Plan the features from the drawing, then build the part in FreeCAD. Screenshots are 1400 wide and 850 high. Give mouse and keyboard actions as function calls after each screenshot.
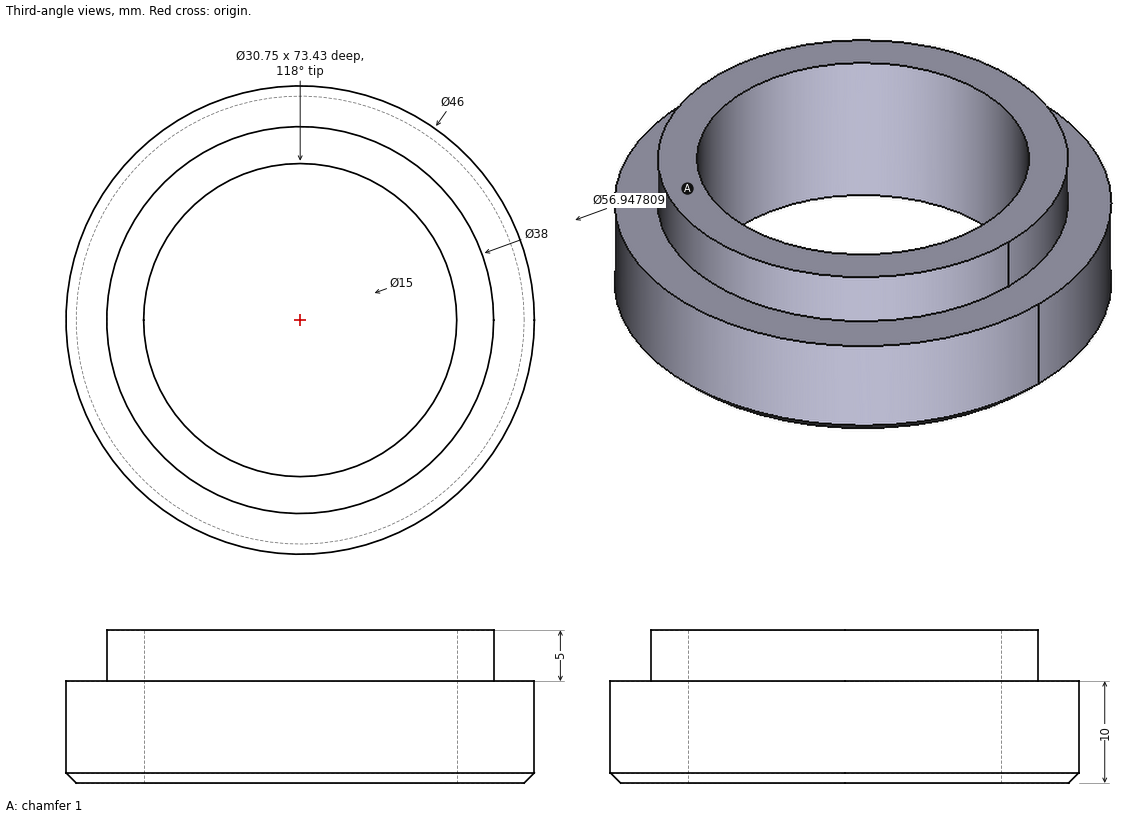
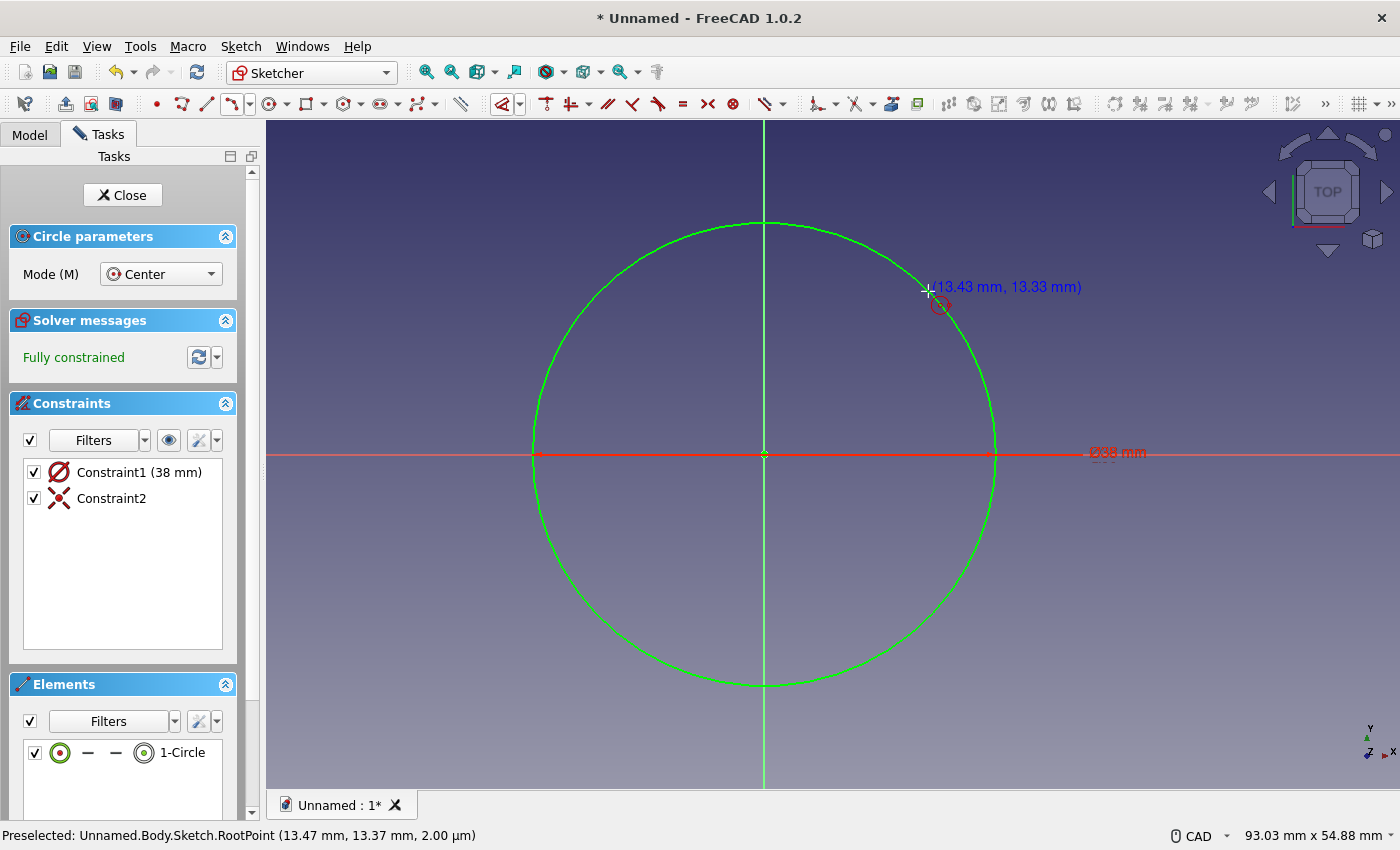
click(764, 454)
move(829, 390)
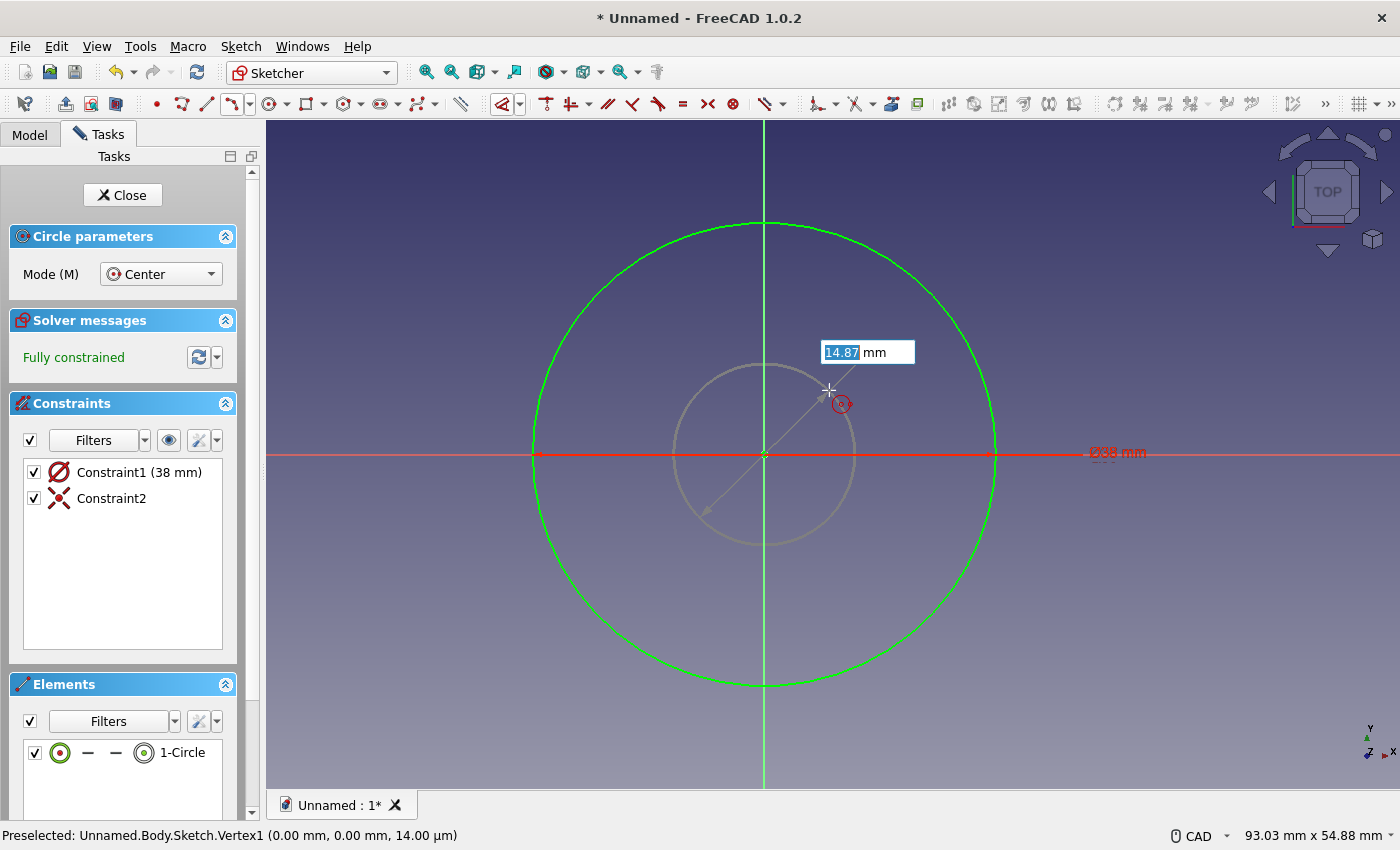
text(15)
key(Return)
key(Escape)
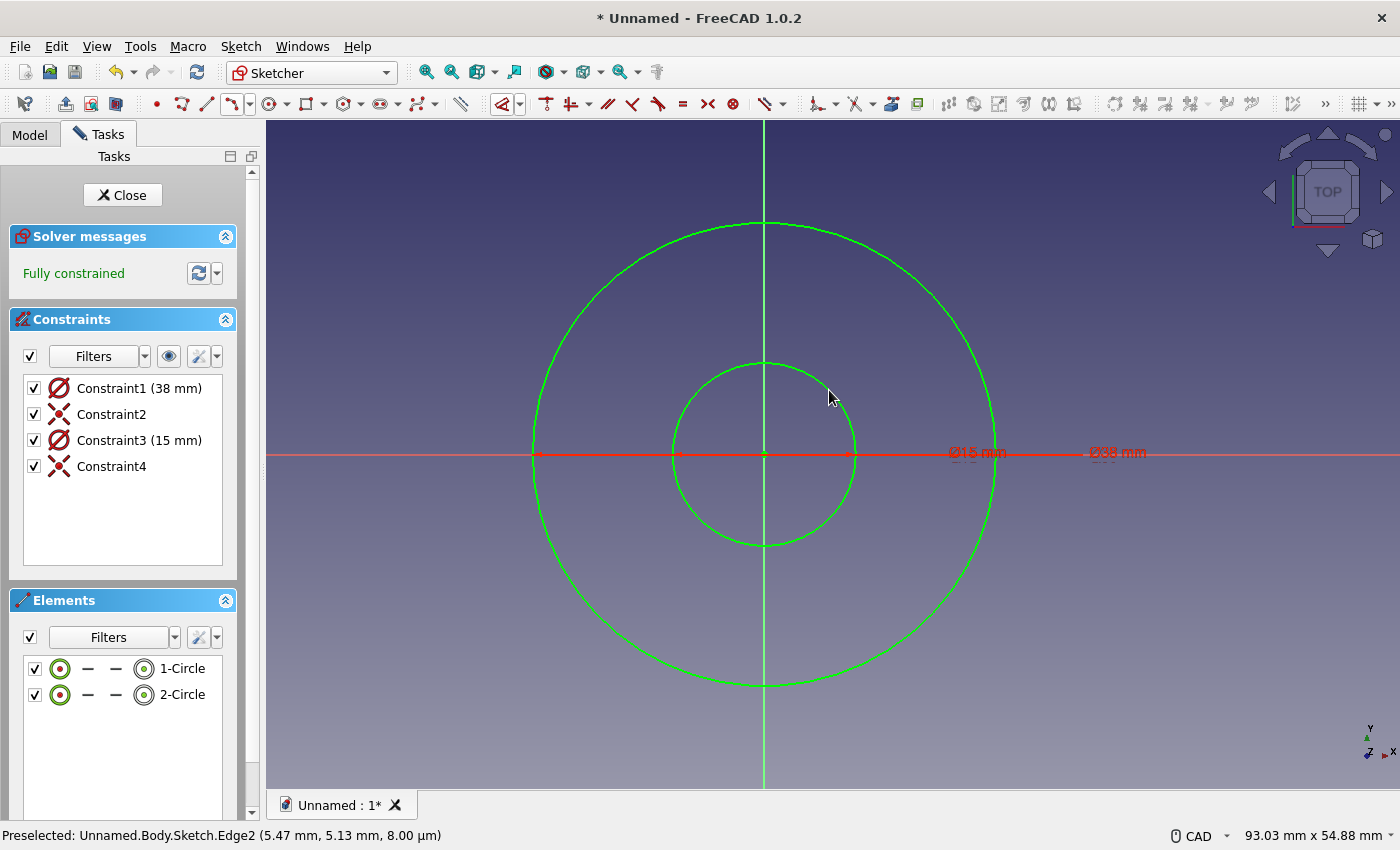
click(123, 195)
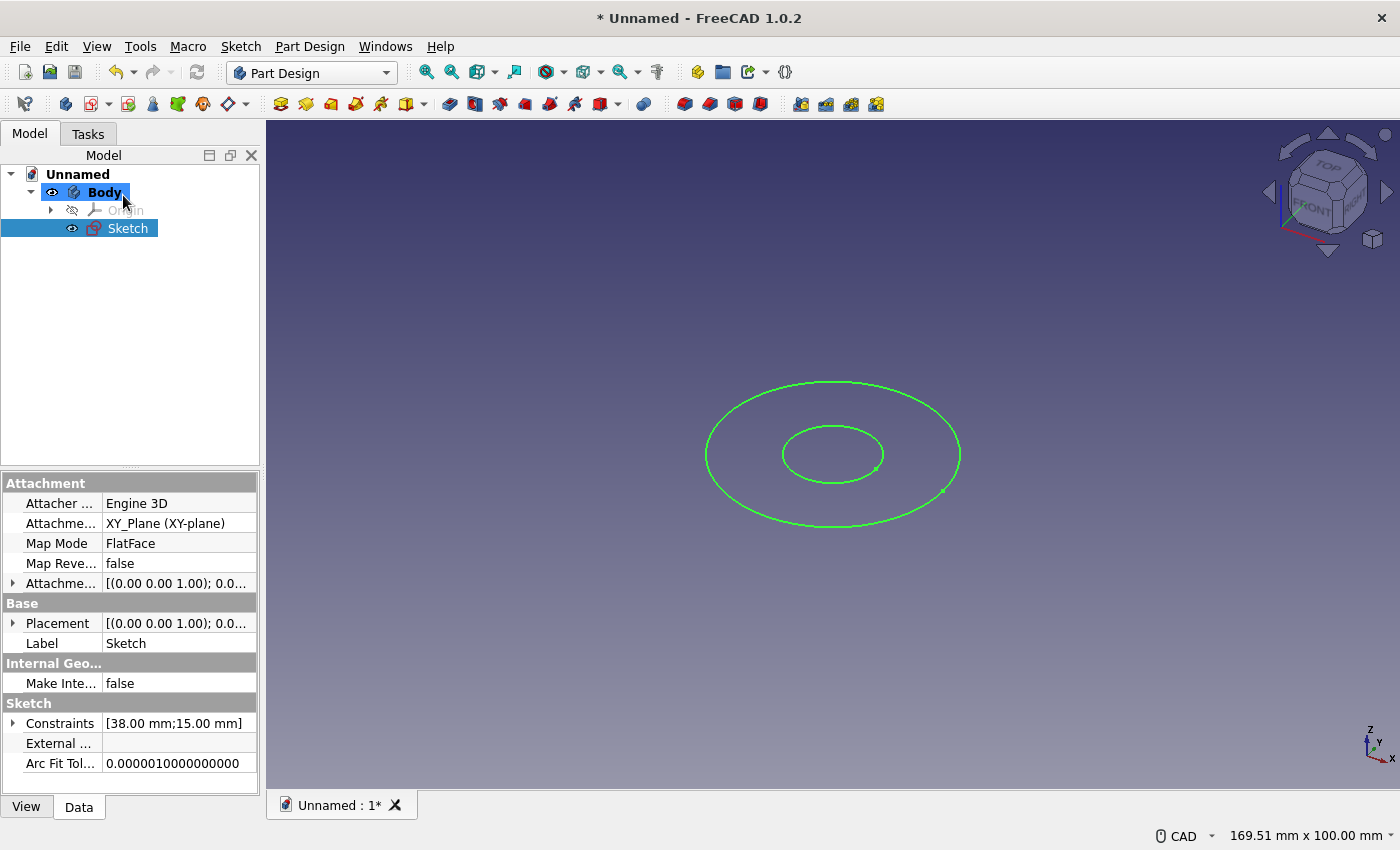
click(281, 104)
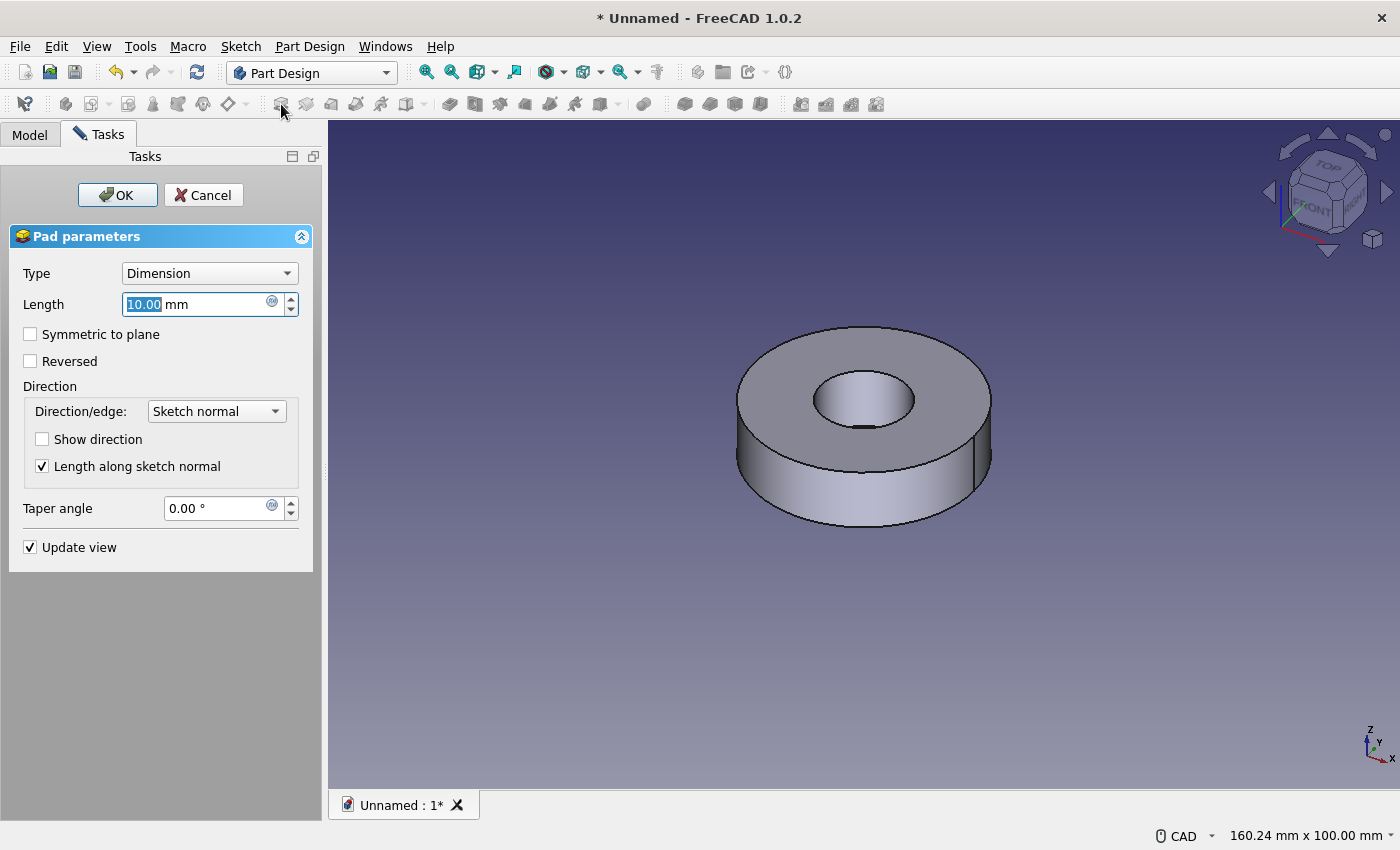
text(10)
key(Tab)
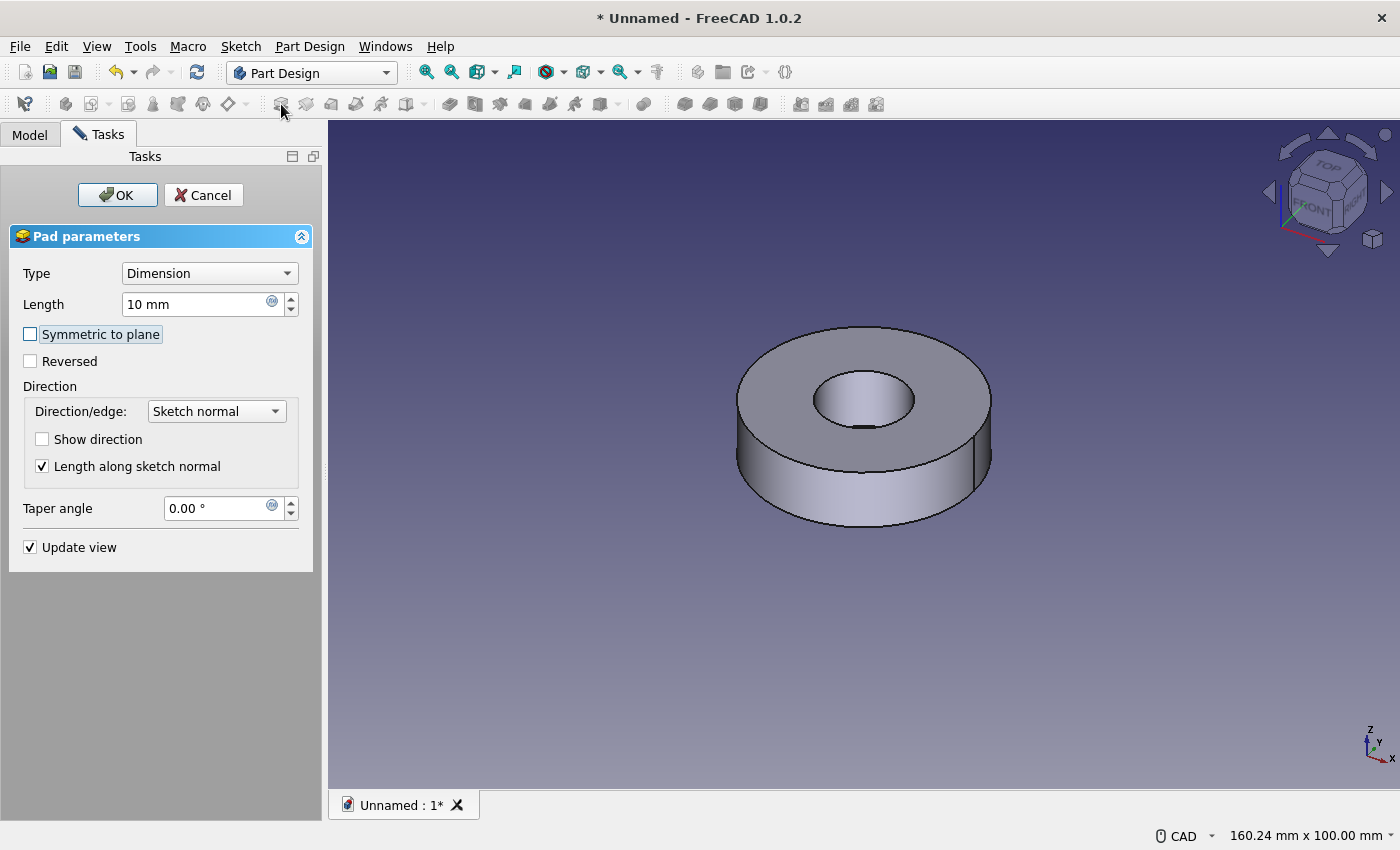
click(118, 195)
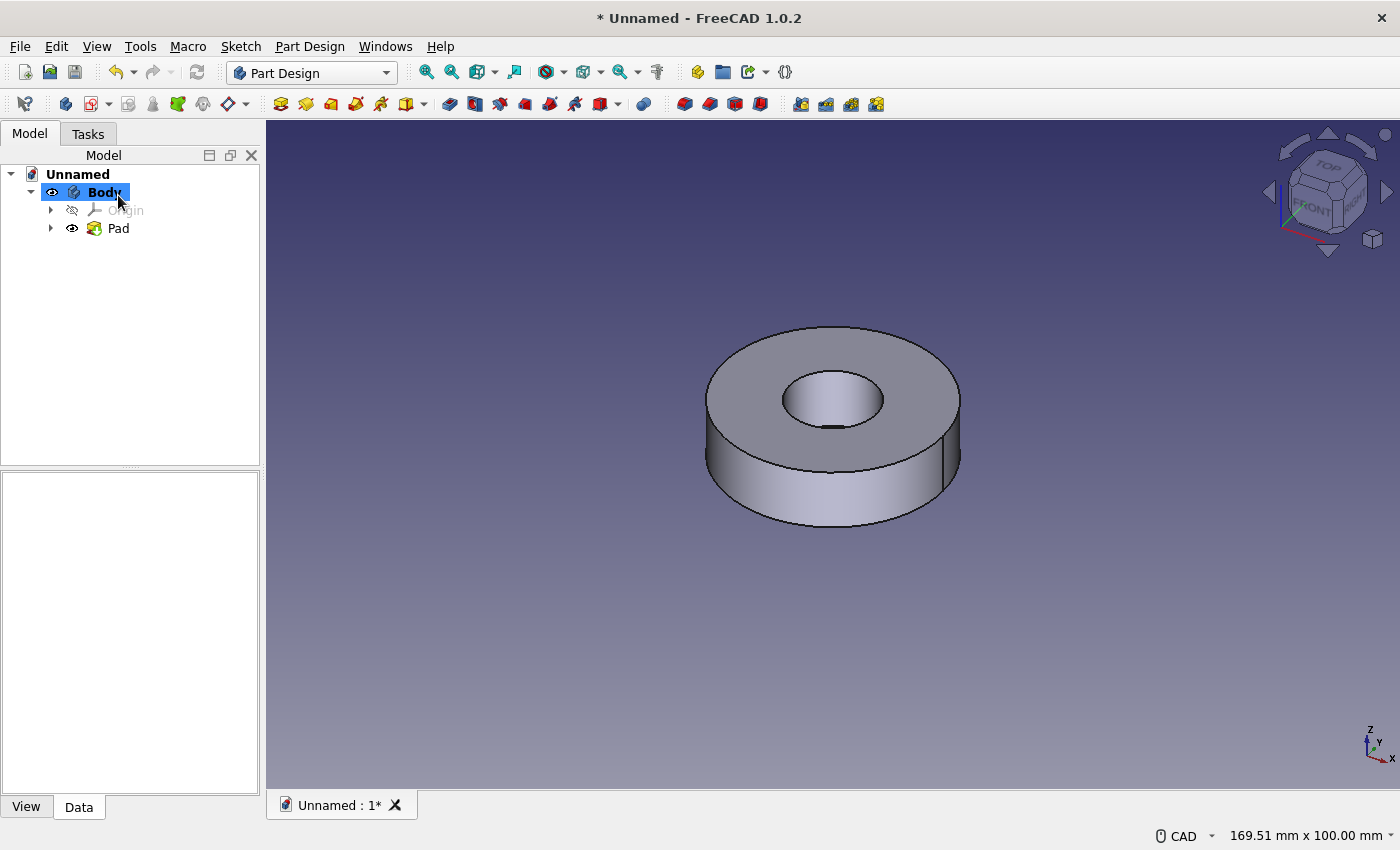
click(427, 72)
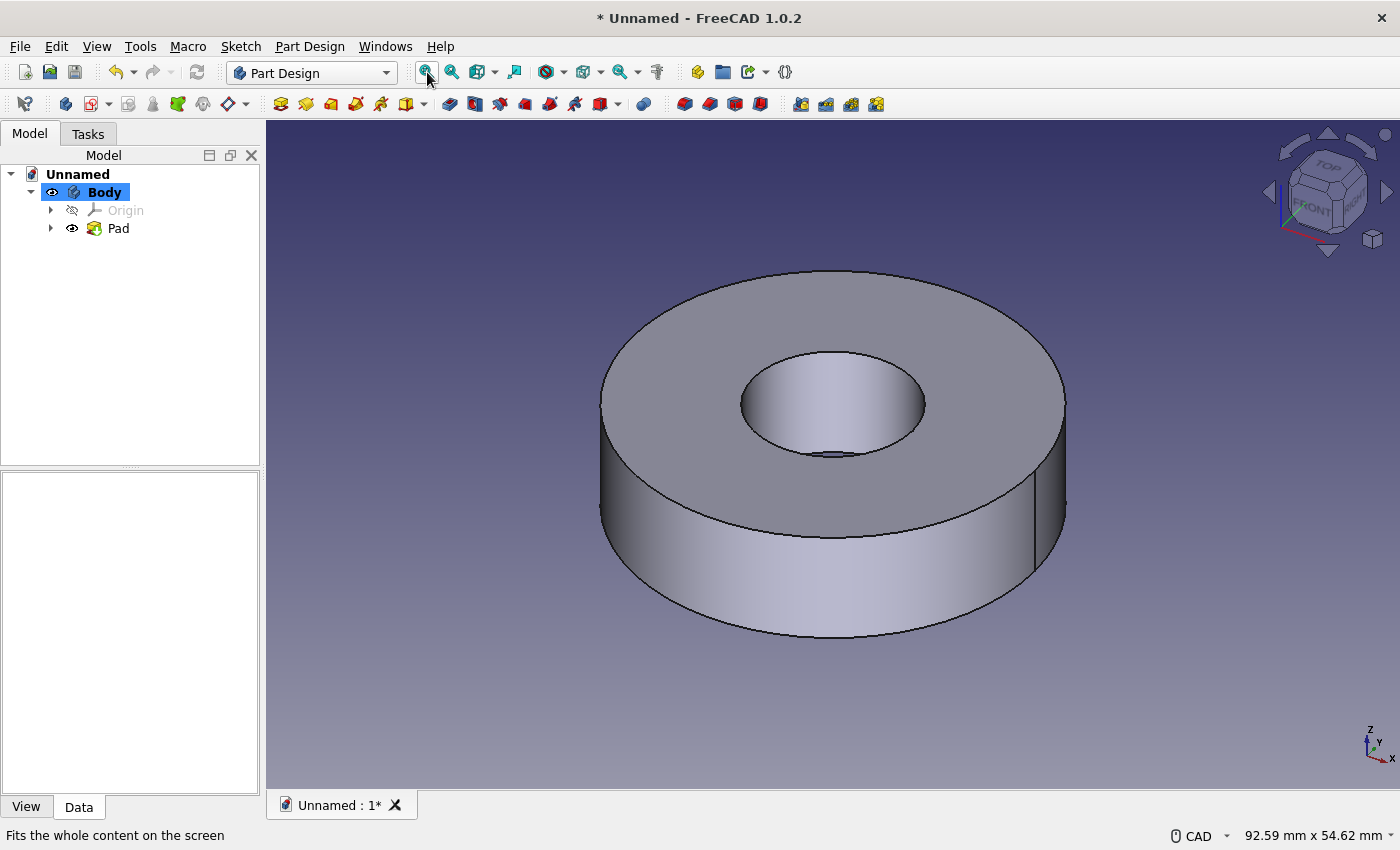
click(842, 318)